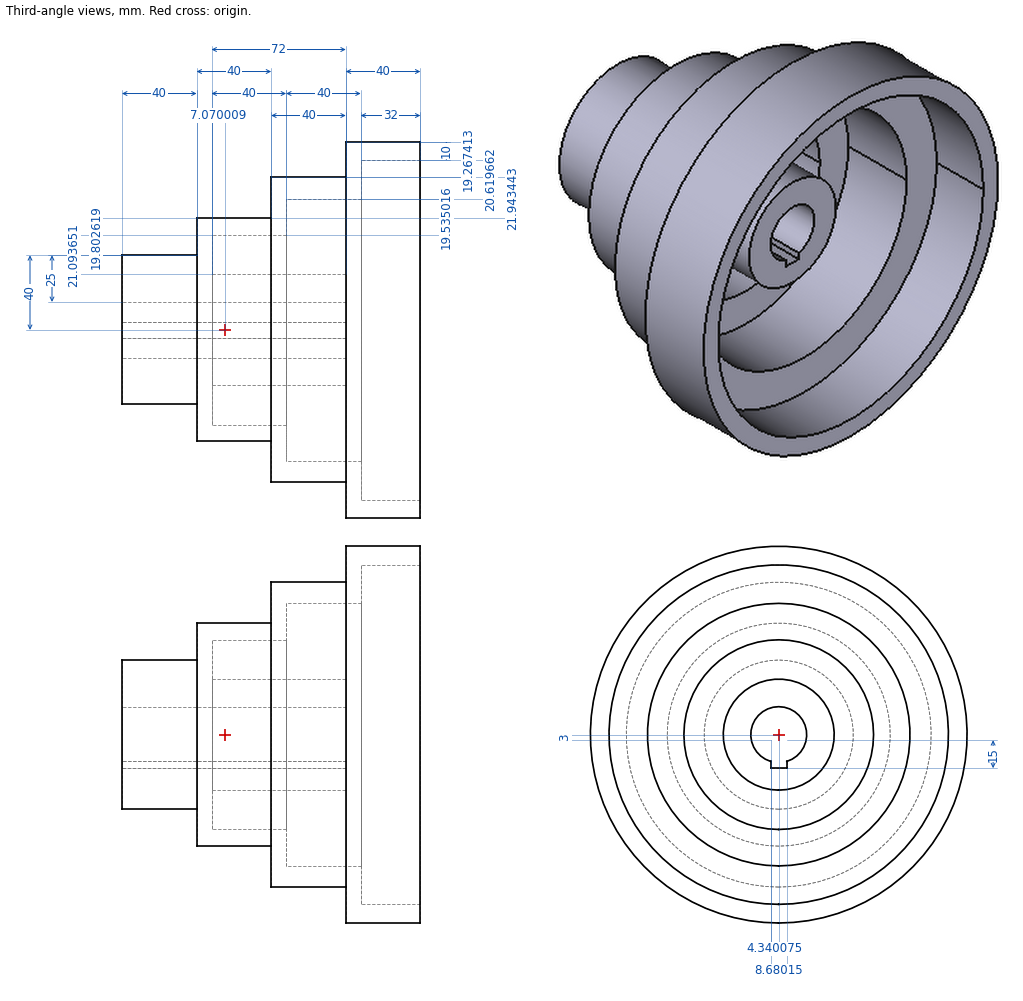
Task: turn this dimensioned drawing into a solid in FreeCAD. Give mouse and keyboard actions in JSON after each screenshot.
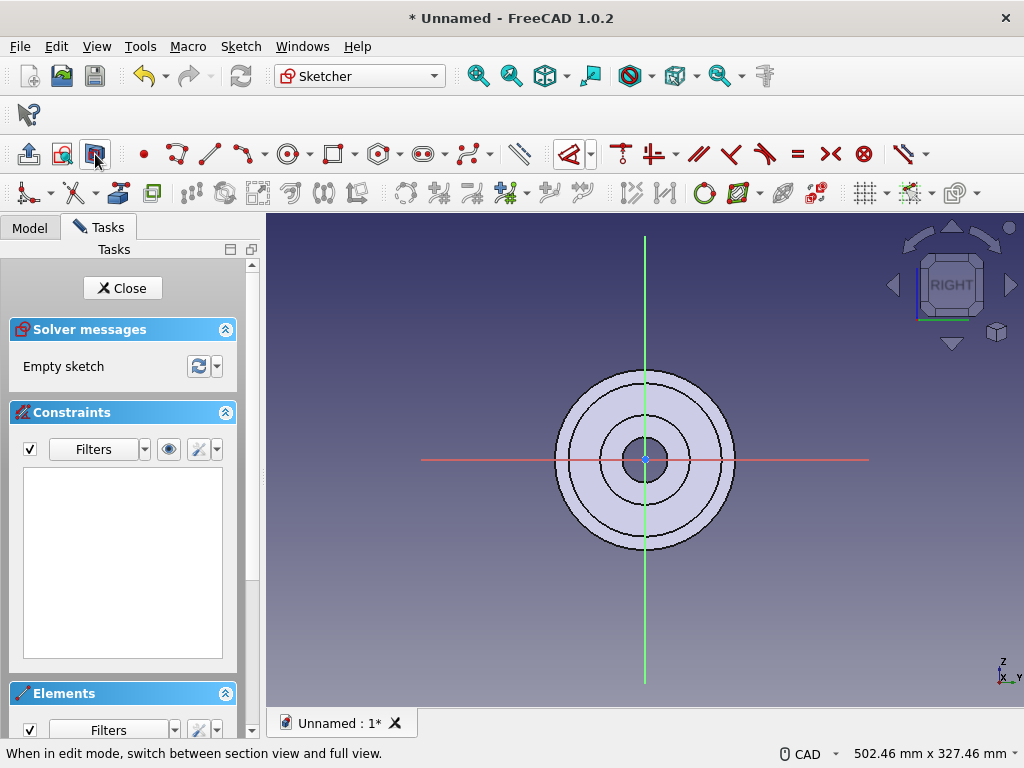
{"action": "scroll", "coordinate": [652, 475], "scroll_direction": "up", "scroll_amount": 12}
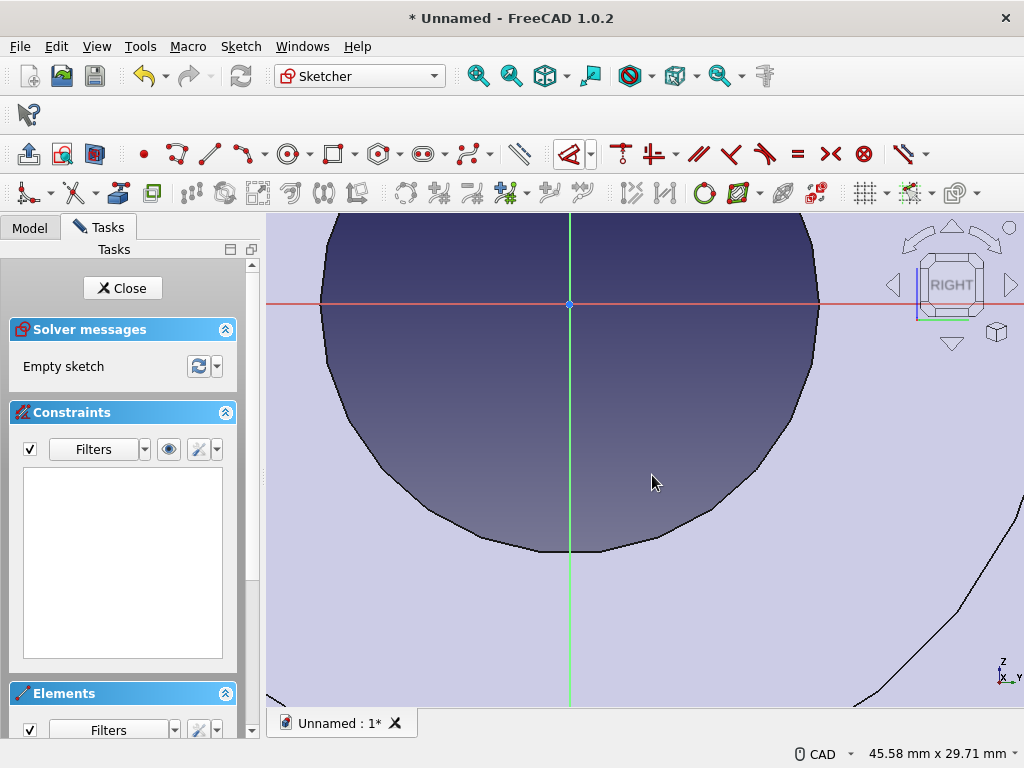
{"action": "left_click", "coordinate": [332, 154]}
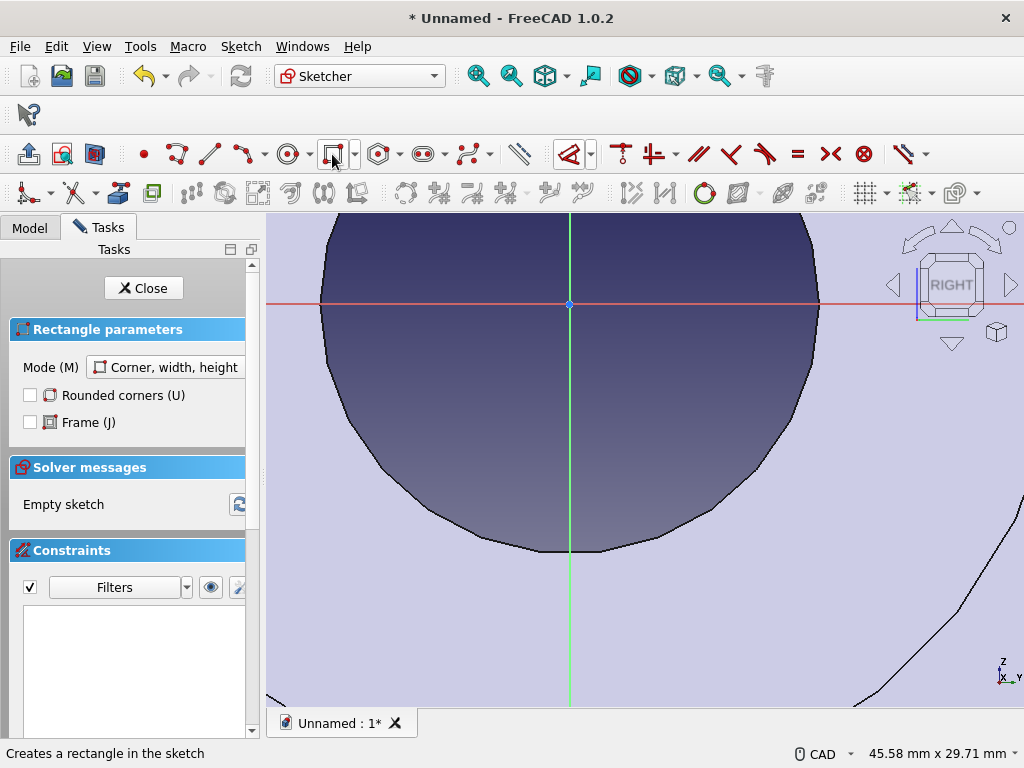
{"action": "left_click", "coordinate": [498, 354]}
{"action": "mouse_move", "coordinate": [642, 604]}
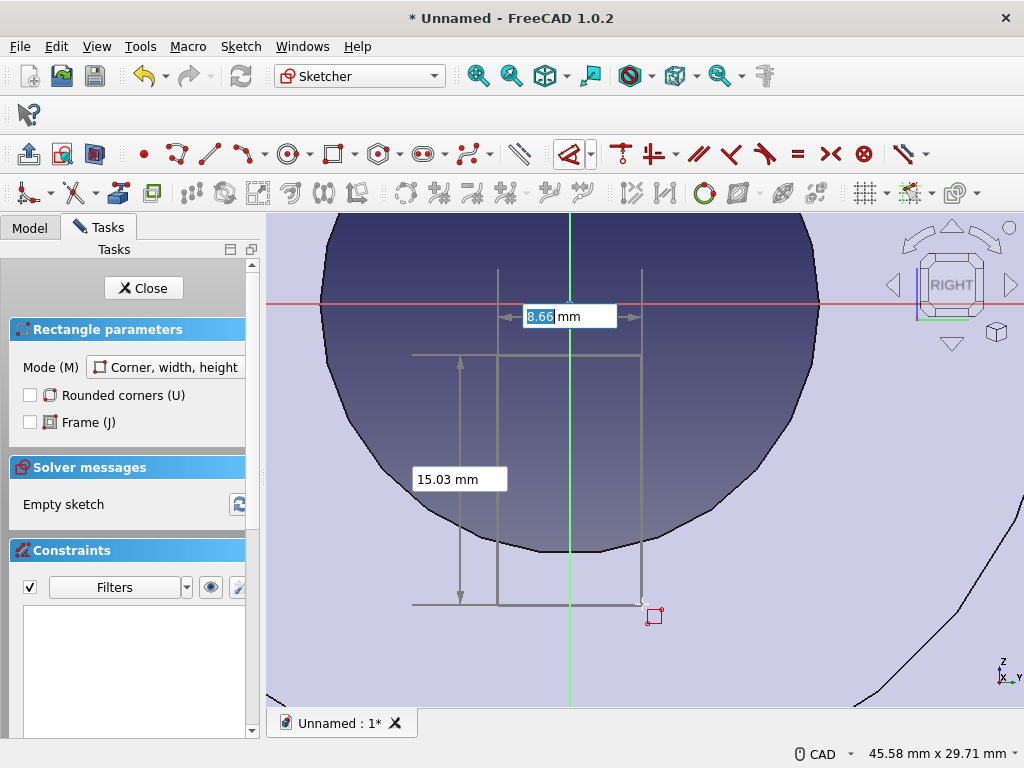
{"action": "type", "text": "8.68015"}
{"action": "key", "text": "Tab"}
{"action": "type", "text": "15"}
{"action": "key", "text": "Return"}
{"action": "key", "text": "Escape"}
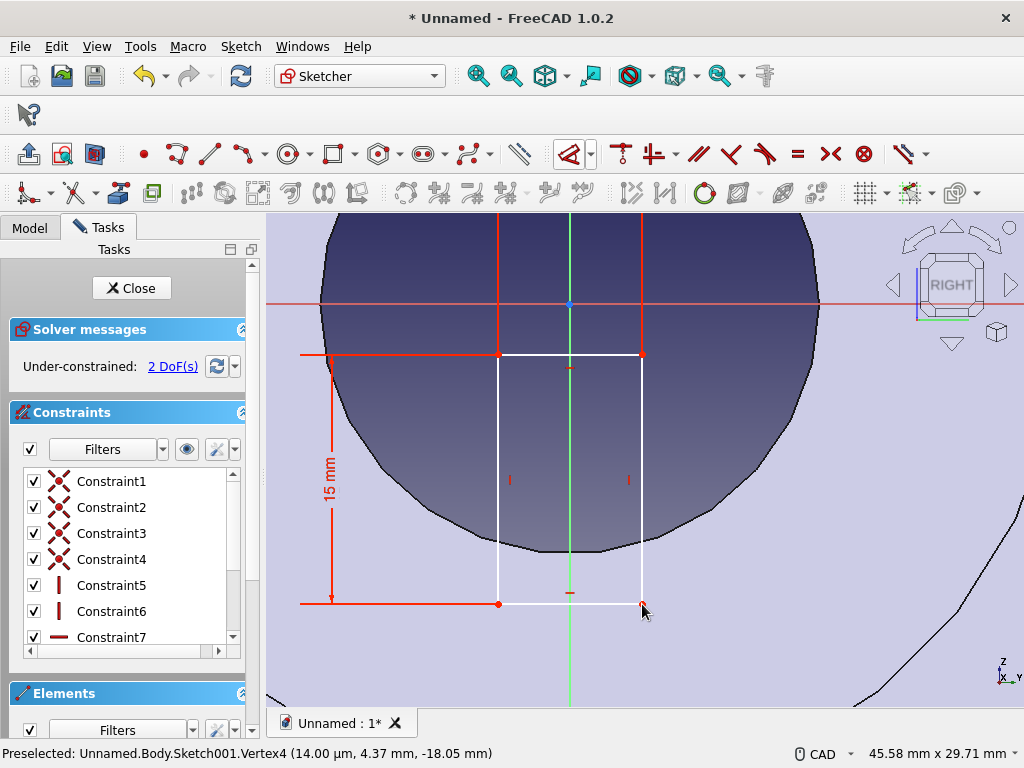
{"action": "left_click", "coordinate": [498, 355]}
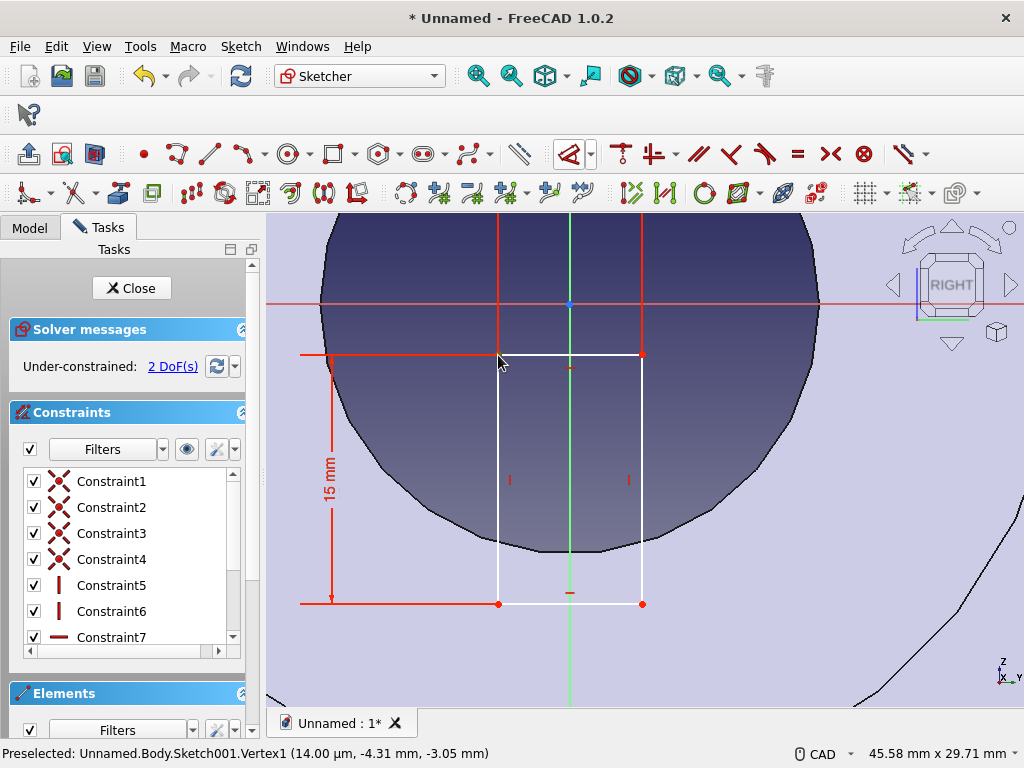
{"action": "left_click", "coordinate": [590, 154]}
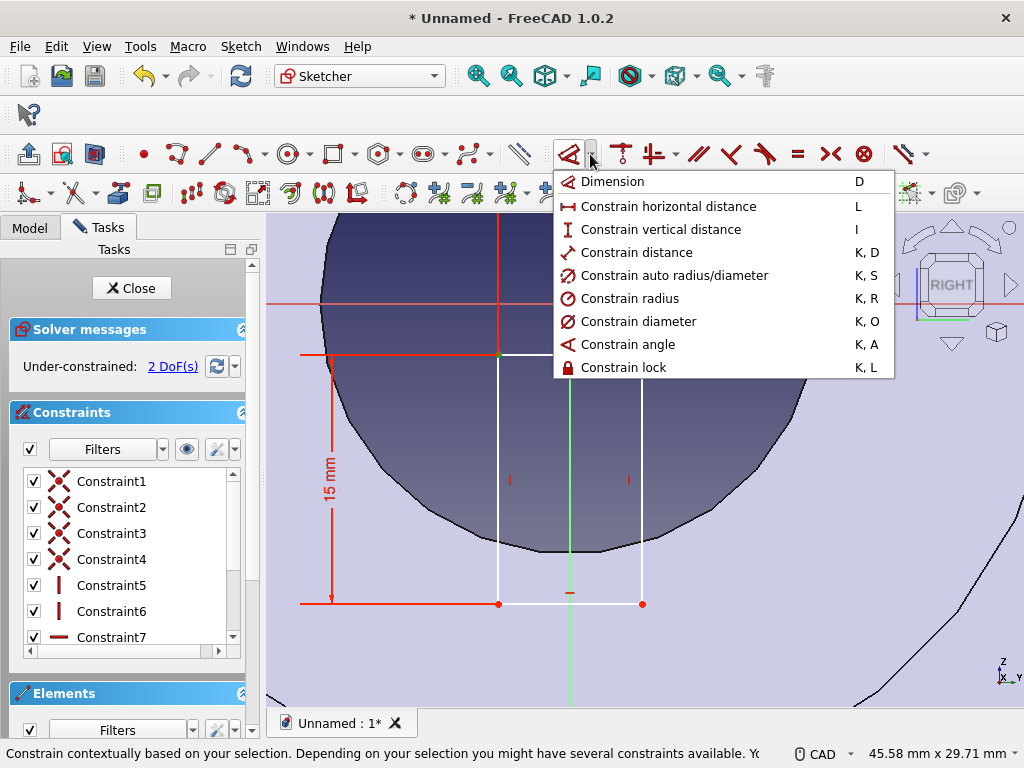
{"action": "left_click", "coordinate": [724, 230]}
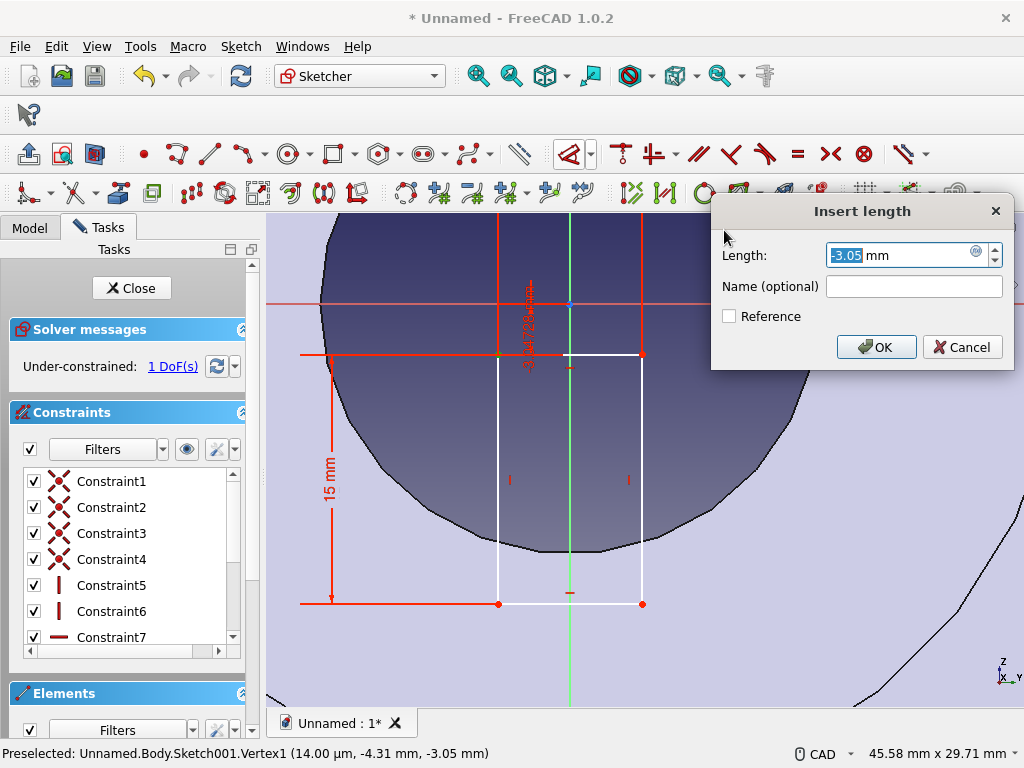
{"action": "type", "text": "-3"}
{"action": "key", "text": "Return"}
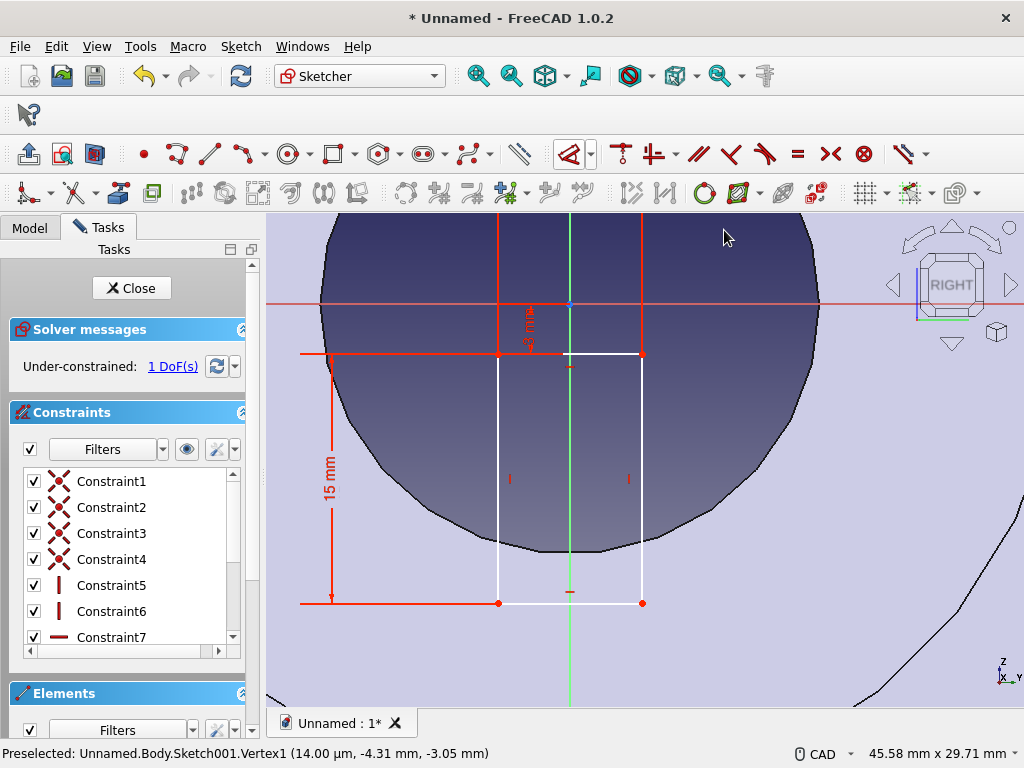
{"action": "left_click", "coordinate": [498, 354]}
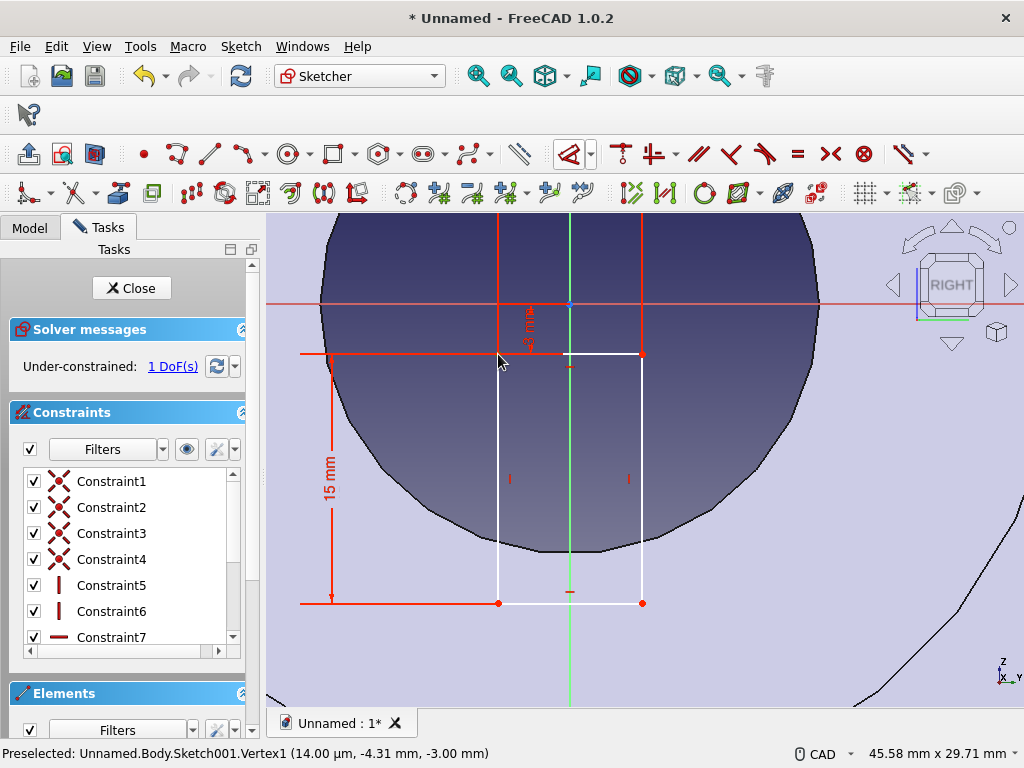
{"action": "left_click", "coordinate": [590, 154]}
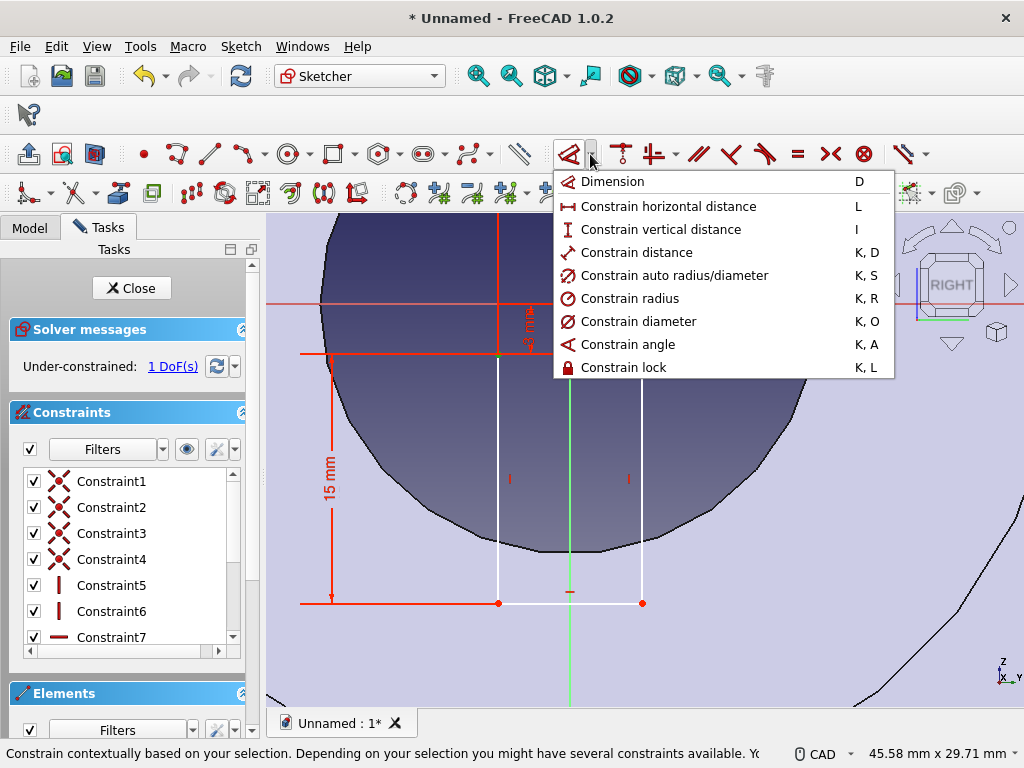
{"action": "left_click", "coordinate": [724, 206]}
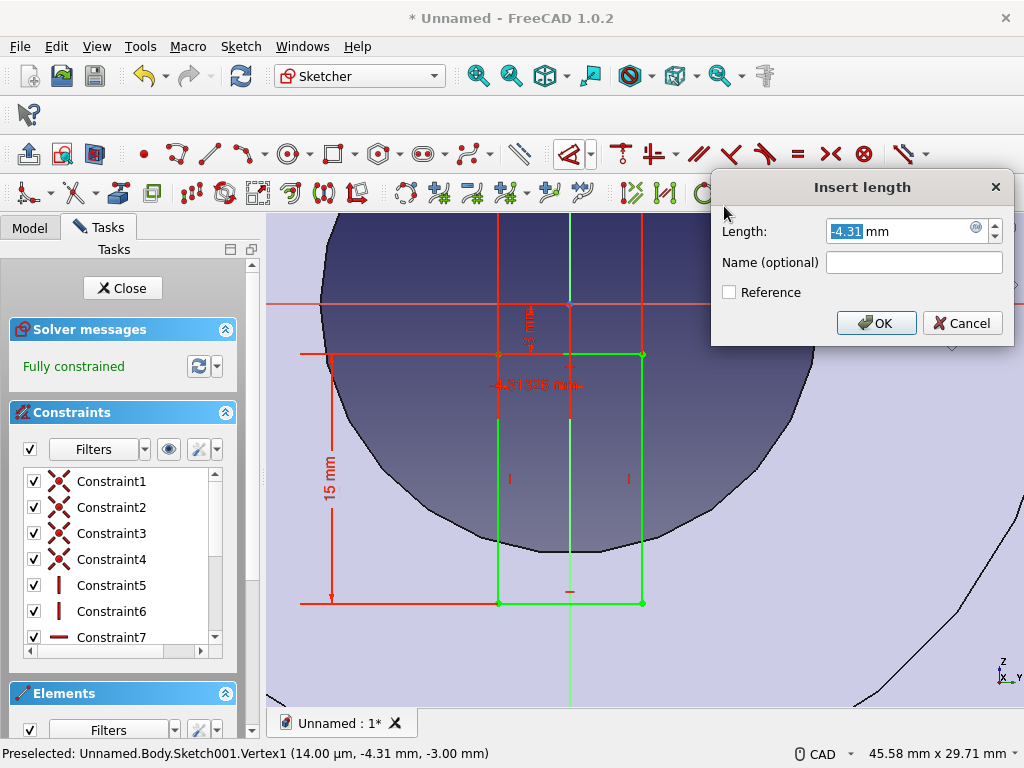
{"action": "type", "text": "-4.340075"}
{"action": "key", "text": "Return"}